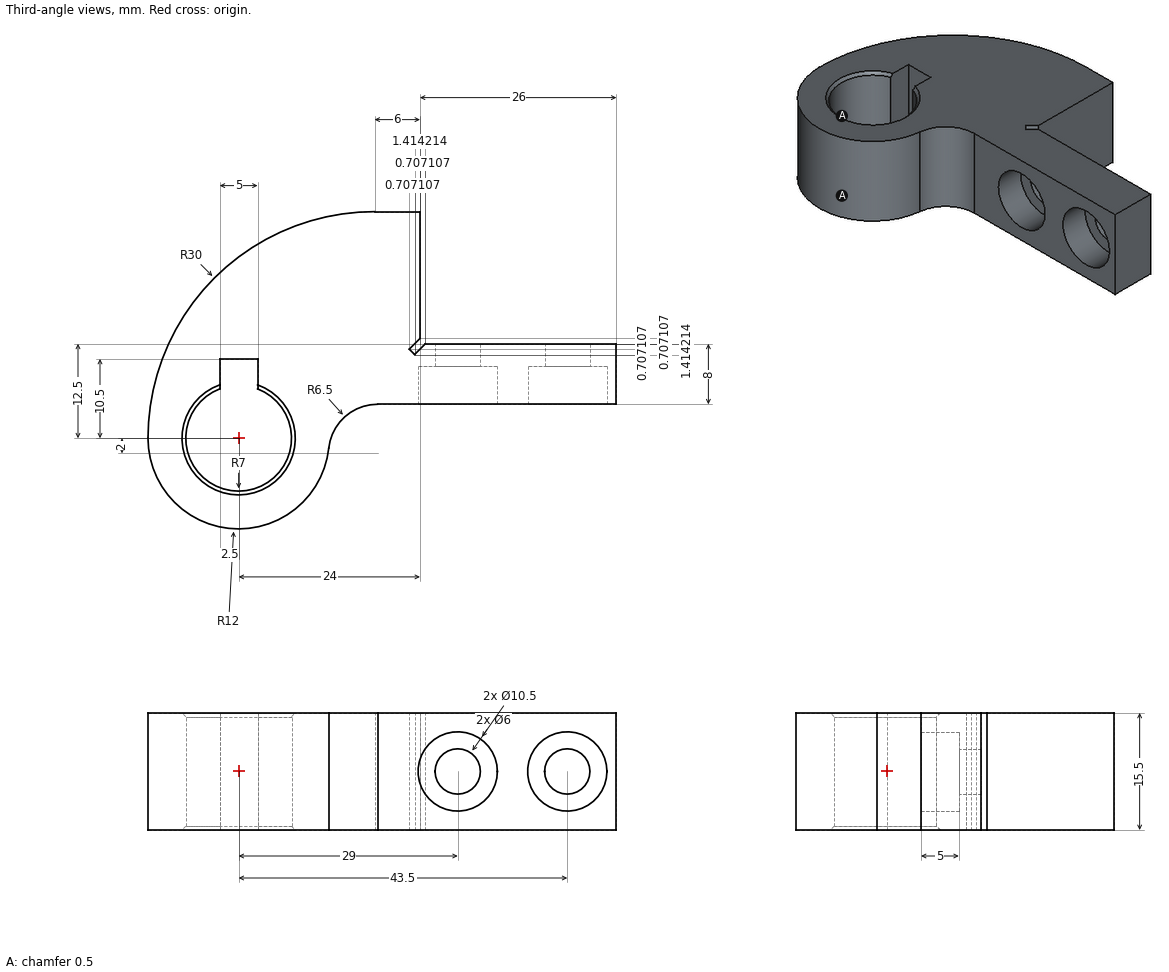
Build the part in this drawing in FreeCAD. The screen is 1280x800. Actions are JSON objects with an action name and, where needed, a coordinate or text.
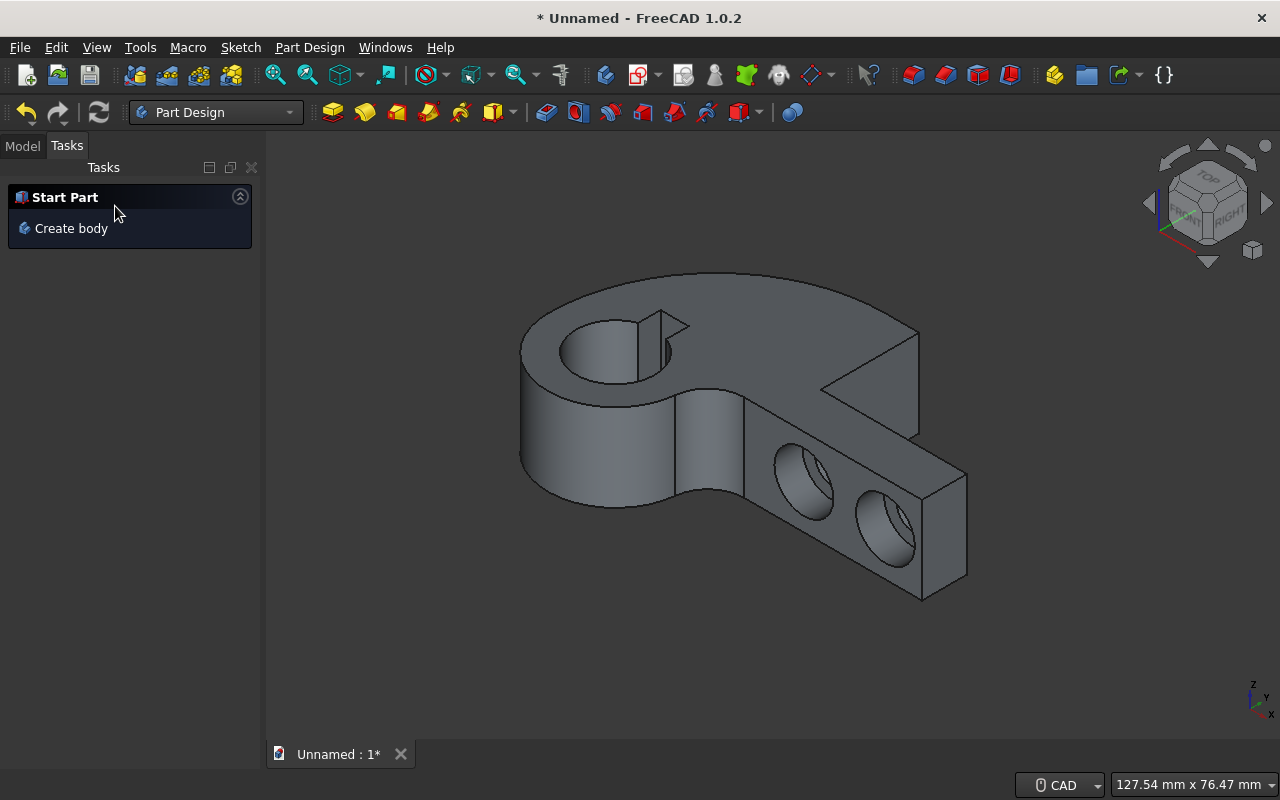
{"action": "left_click", "coordinate": [757, 335]}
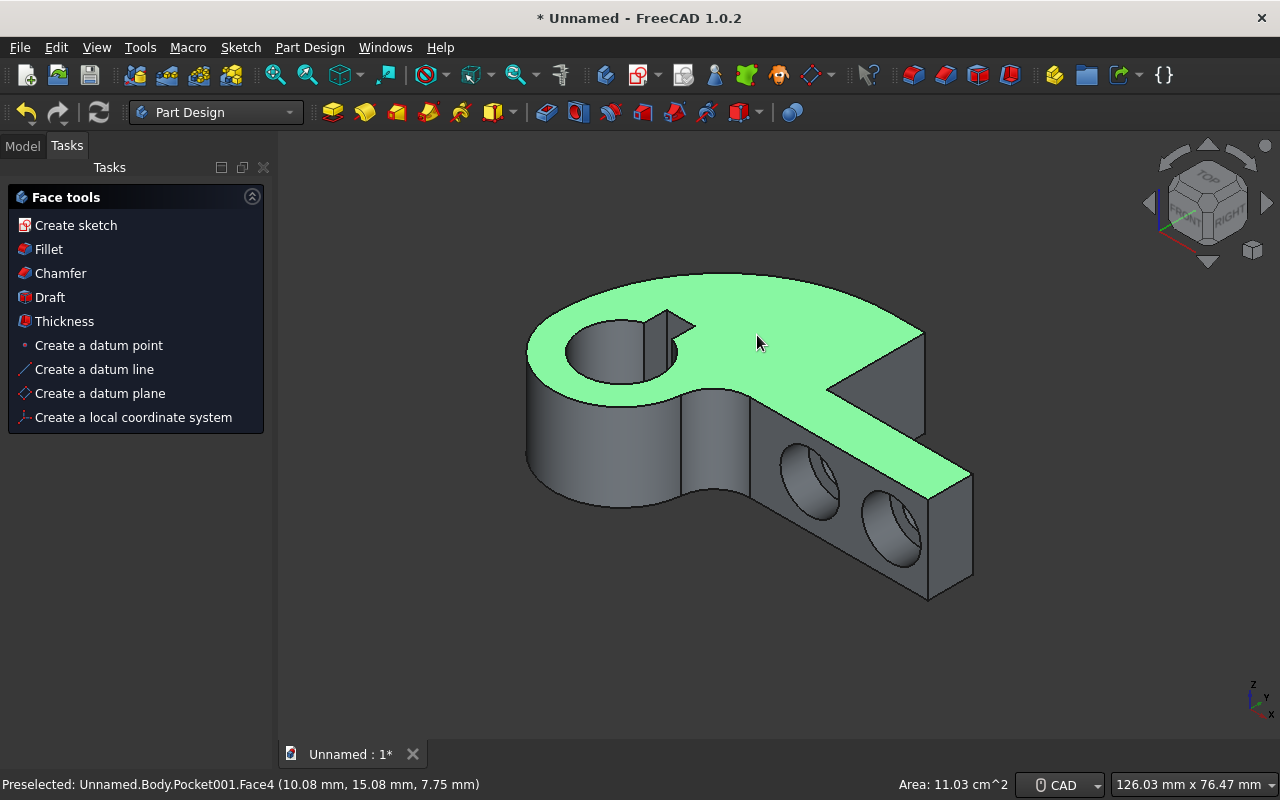
{"action": "left_click", "coordinate": [638, 76]}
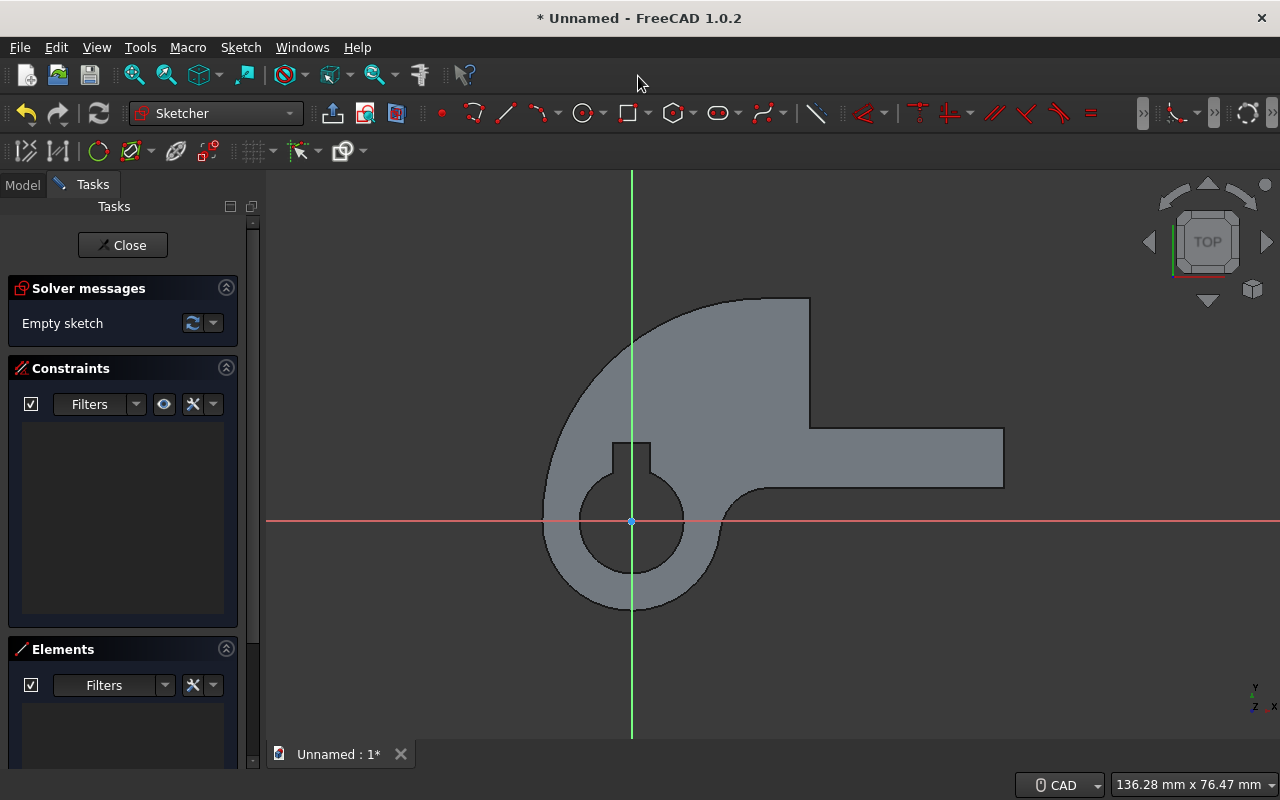
{"action": "scroll", "coordinate": [813, 430], "scroll_direction": "up", "scroll_amount": 15}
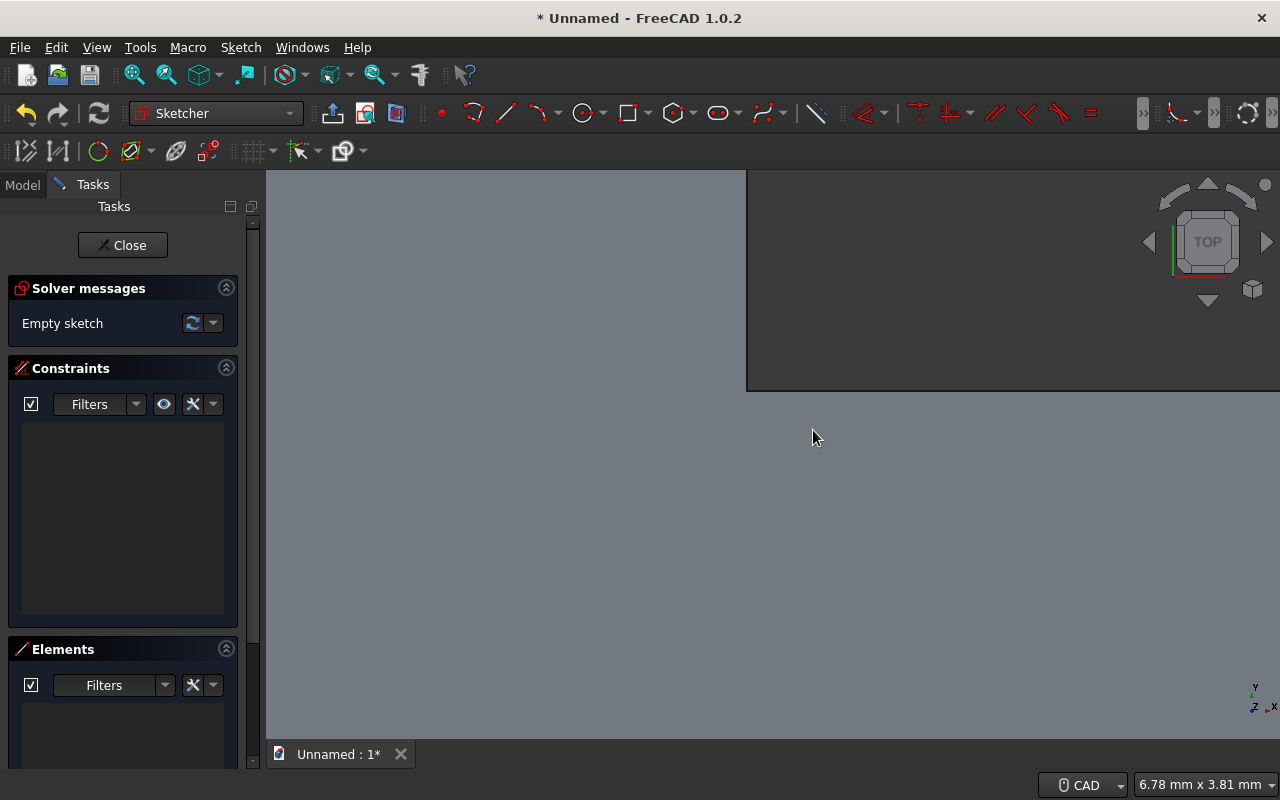
{"action": "key", "text": "g m"}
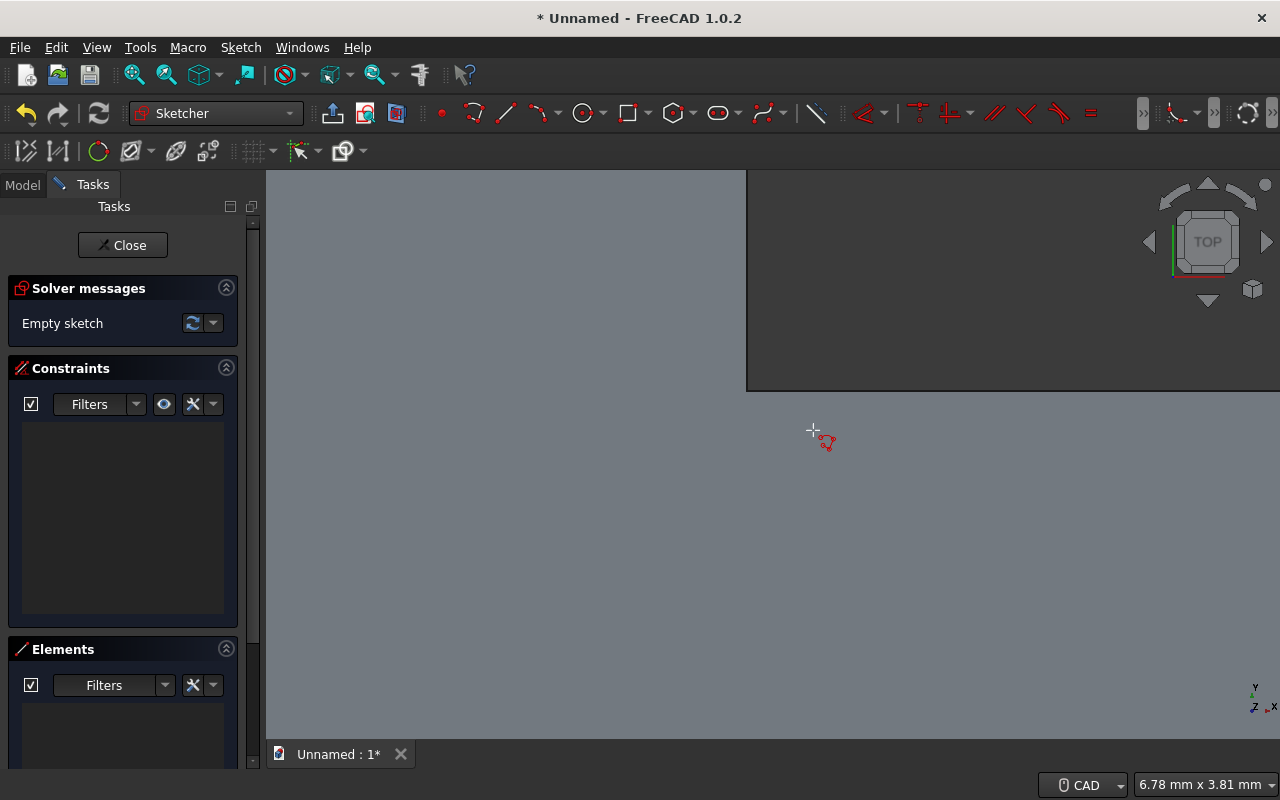
{"action": "left_click", "coordinate": [535, 496]}
{"action": "left_click", "coordinate": [641, 602]}
{"action": "left_click", "coordinate": [852, 391]}
{"action": "left_click", "coordinate": [747, 285]}
{"action": "left_click", "coordinate": [535, 497]}
{"action": "key", "text": "Escape"}
{"action": "key", "text": "Escape"}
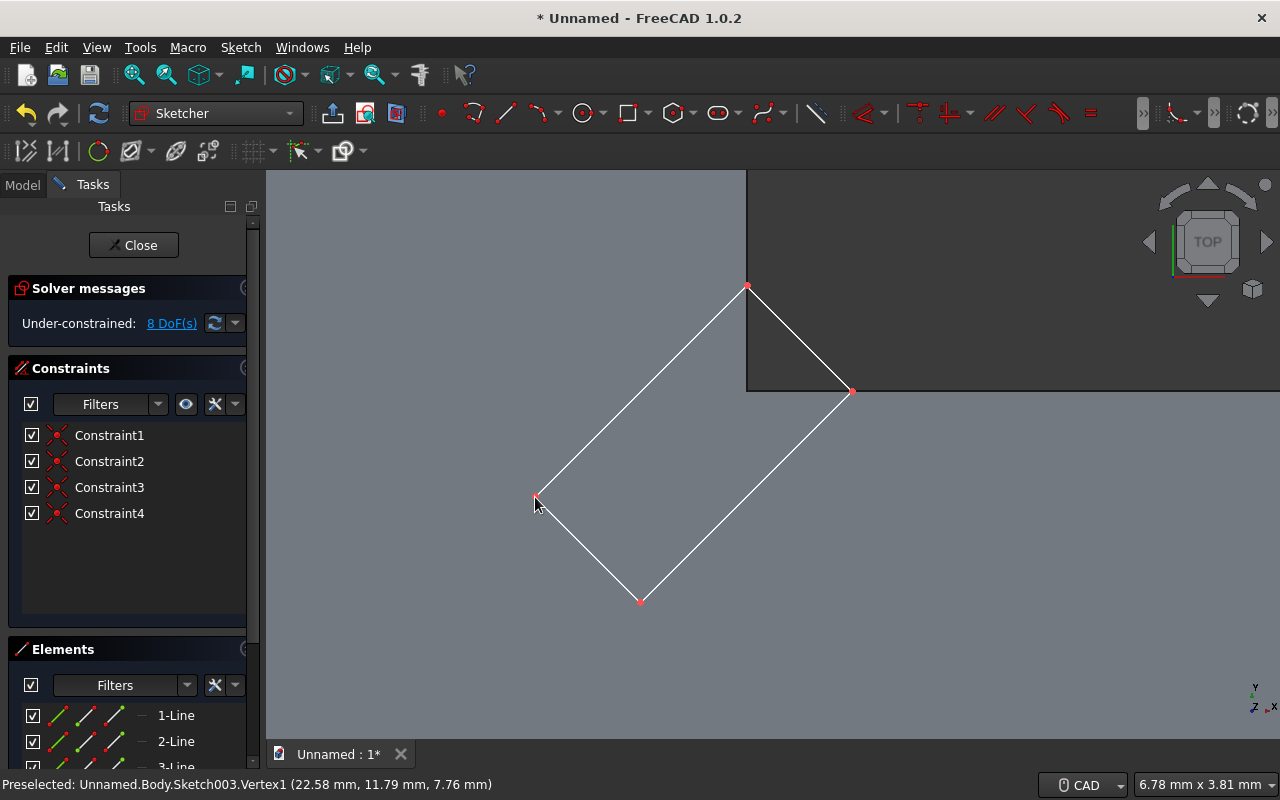
{"action": "left_click", "coordinate": [864, 114]}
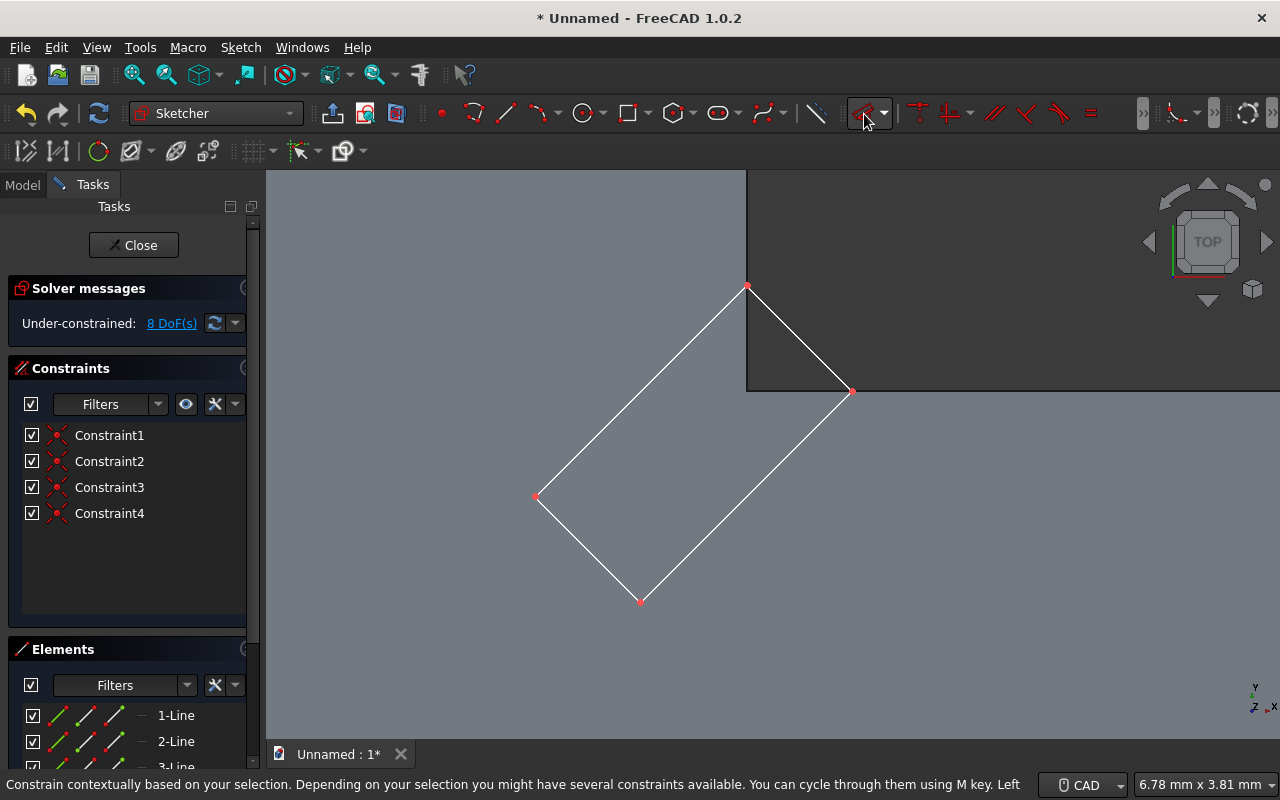
{"action": "left_click", "coordinate": [747, 286]}
{"action": "left_click", "coordinate": [521, 252]}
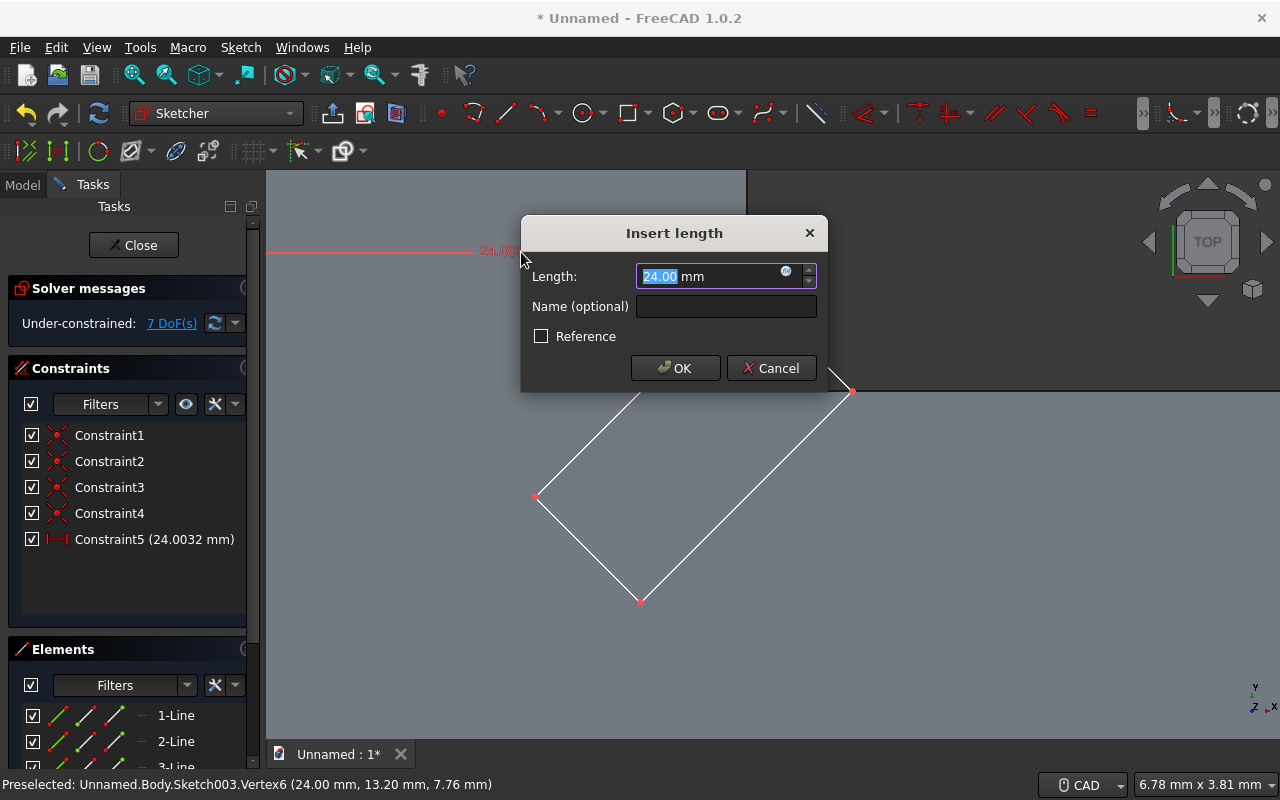
{"action": "type", "text": "24"}
{"action": "key", "text": "Return"}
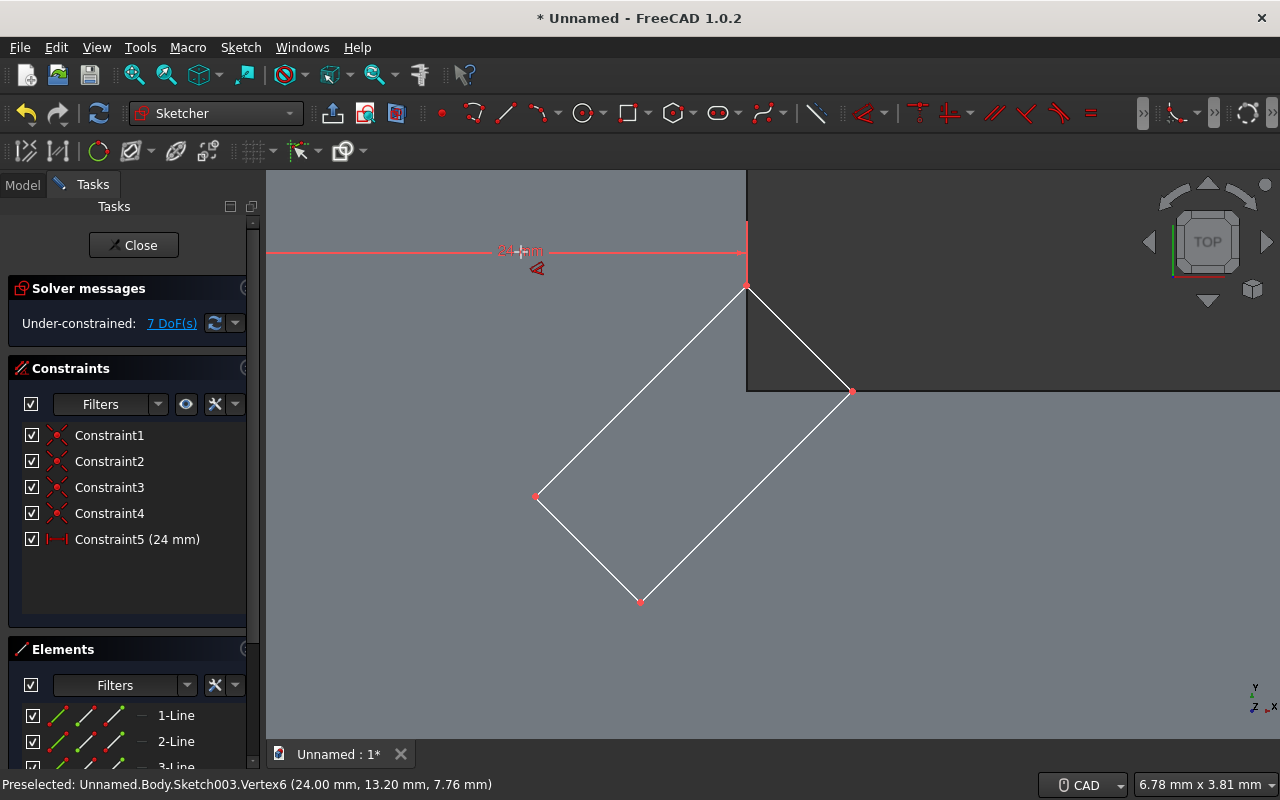
{"action": "left_click", "coordinate": [852, 392]}
{"action": "left_click", "coordinate": [886, 551]}